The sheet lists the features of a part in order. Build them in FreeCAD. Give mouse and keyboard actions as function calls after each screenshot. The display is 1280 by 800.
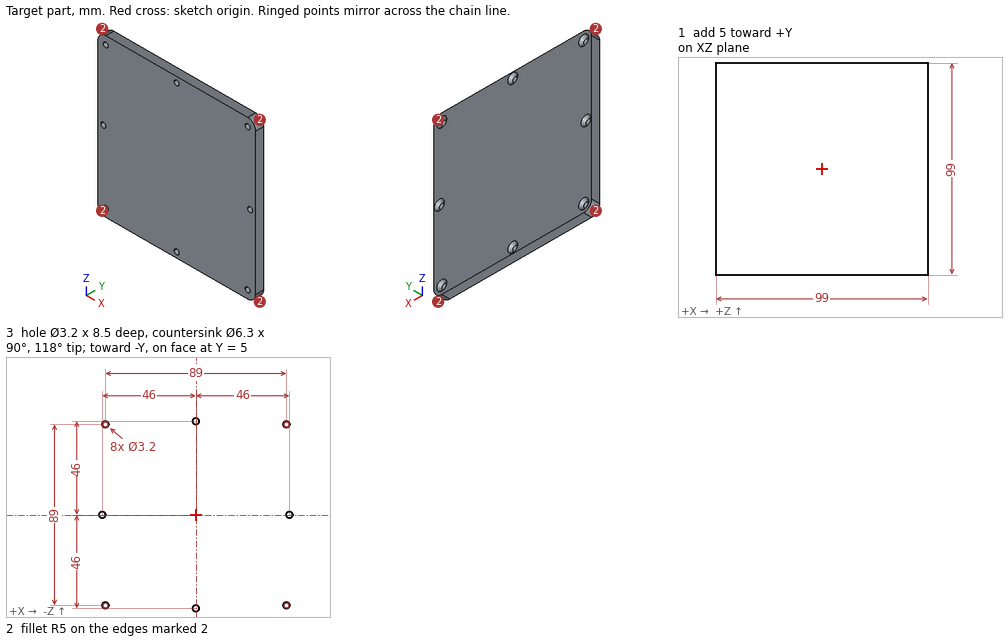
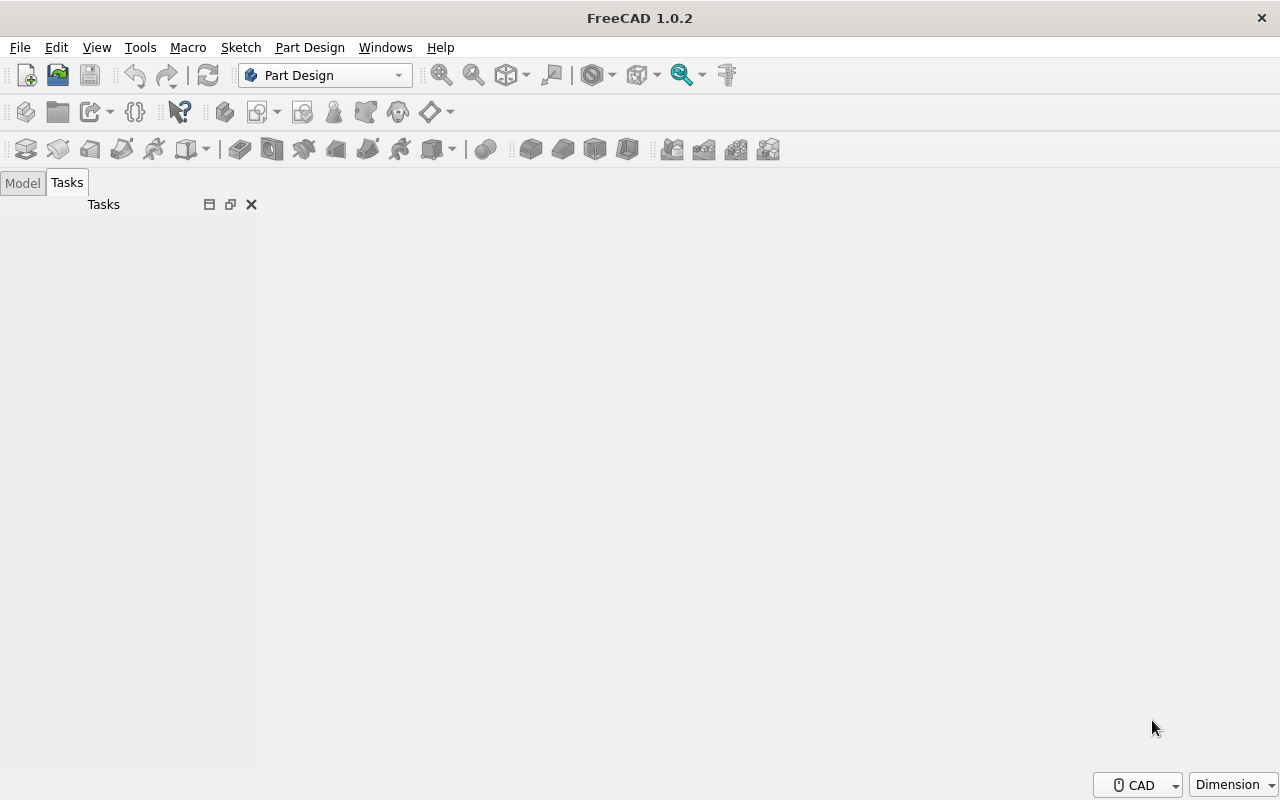
click(26, 76)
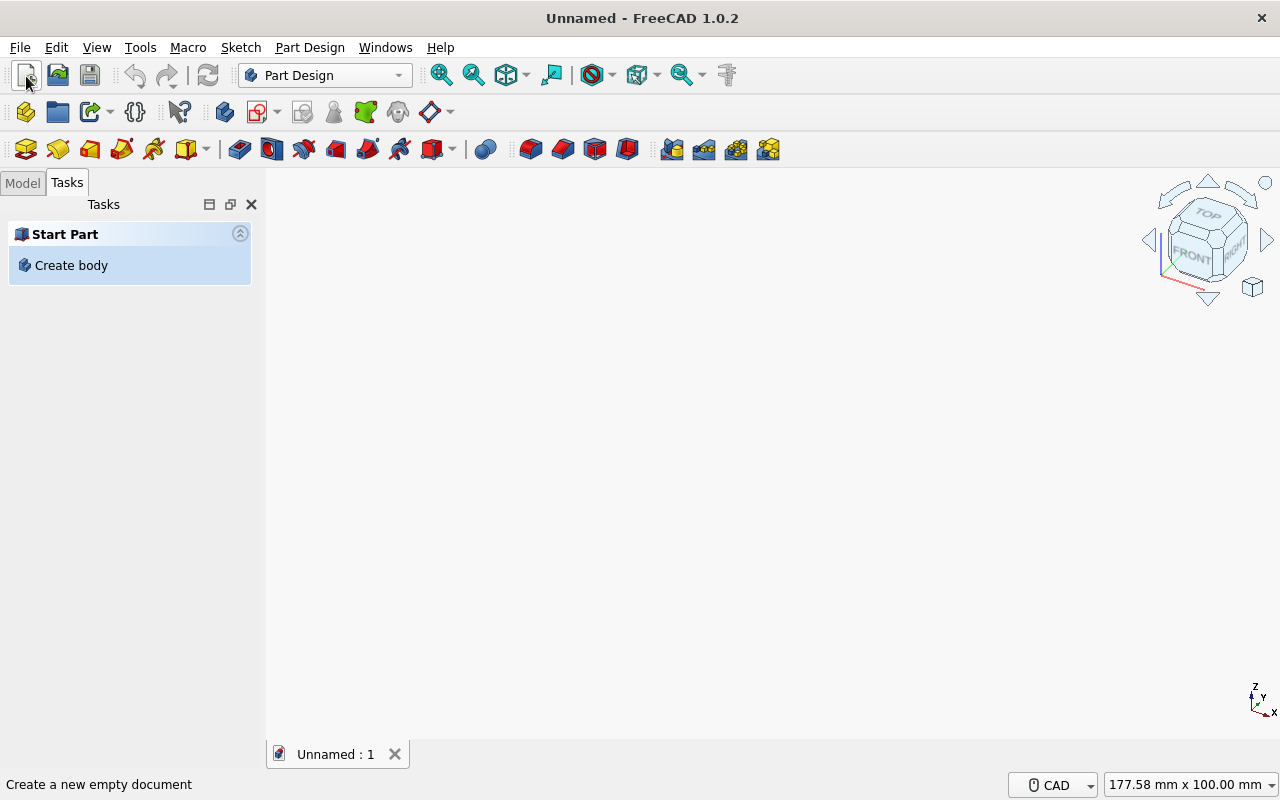
click(258, 112)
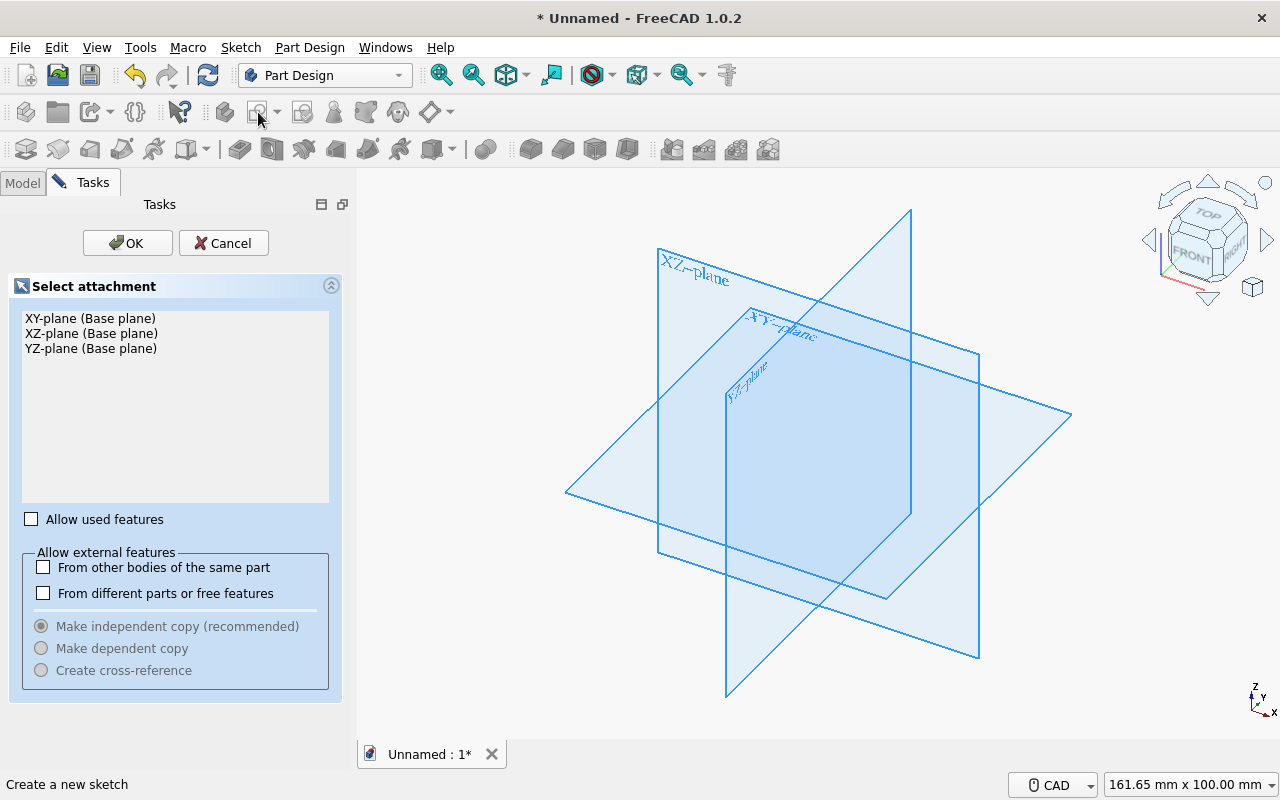
click(82, 334)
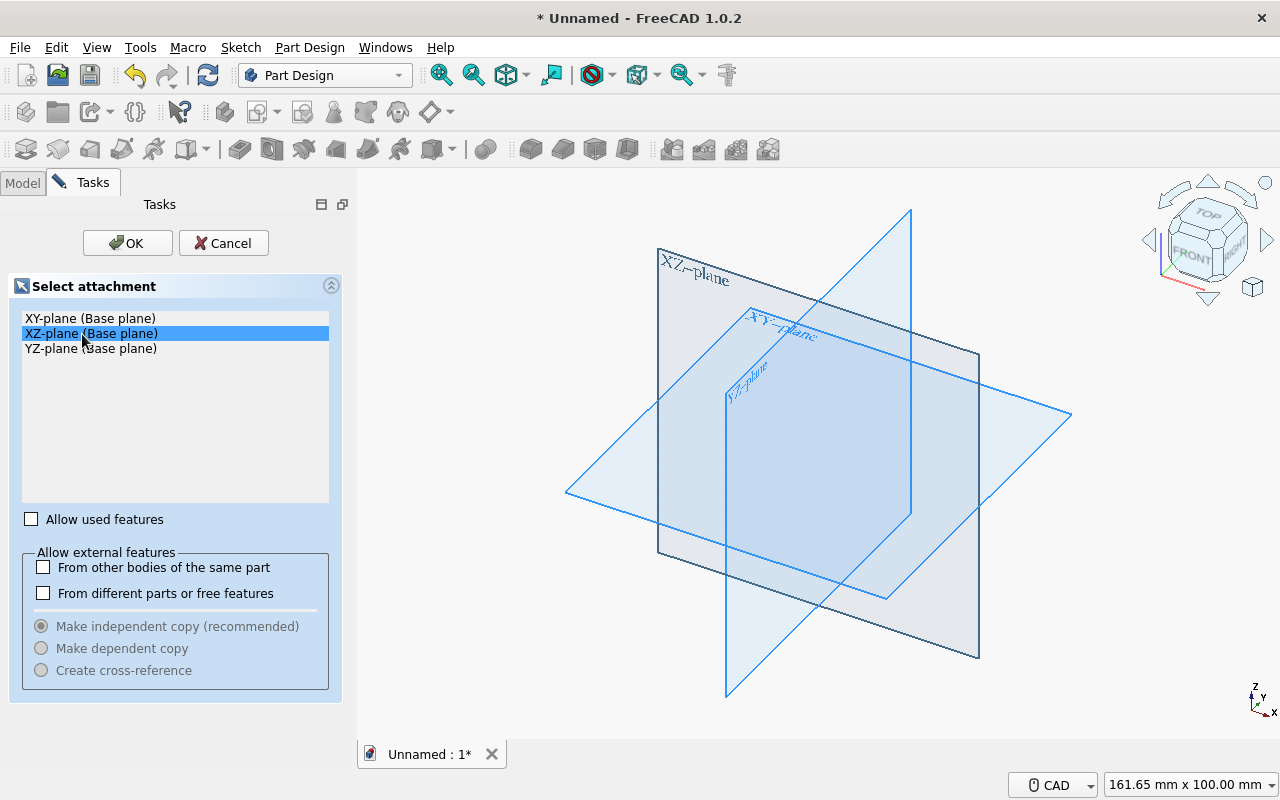
click(128, 243)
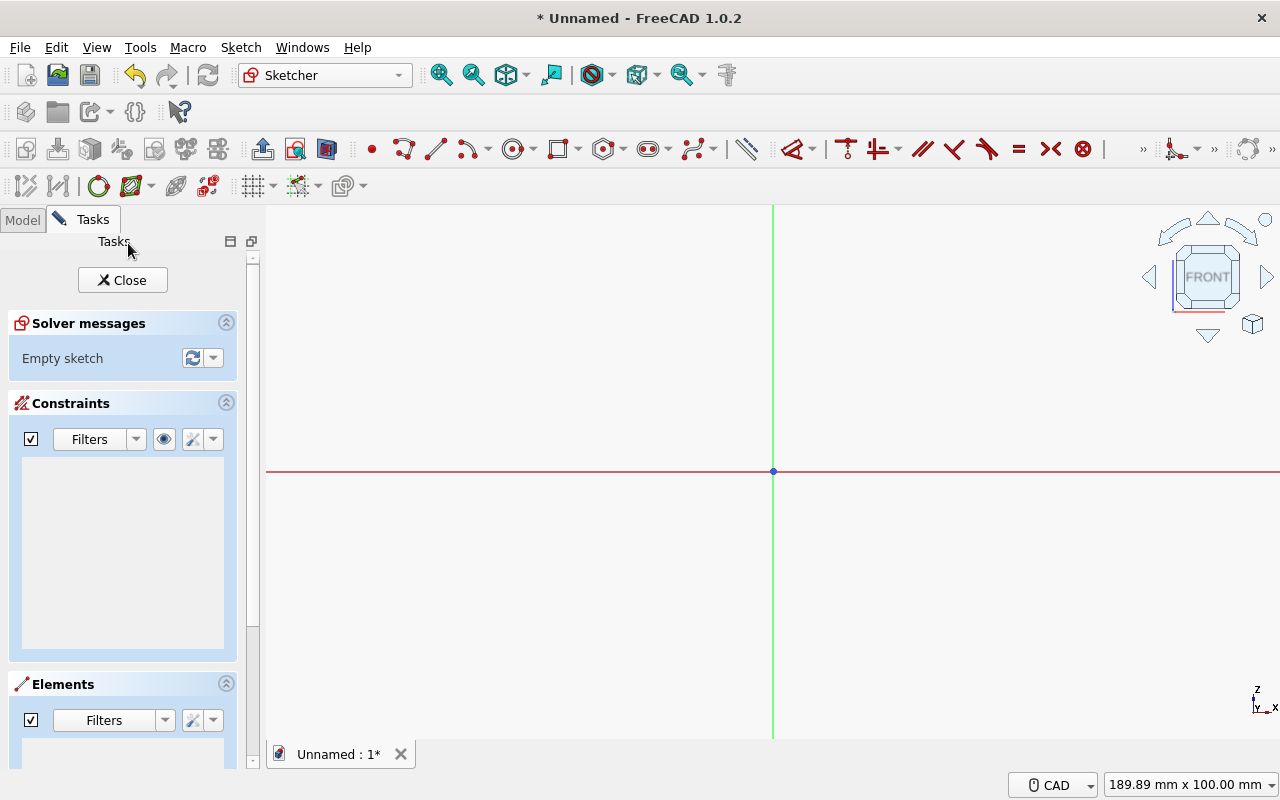
scroll(565, 472, down, 2)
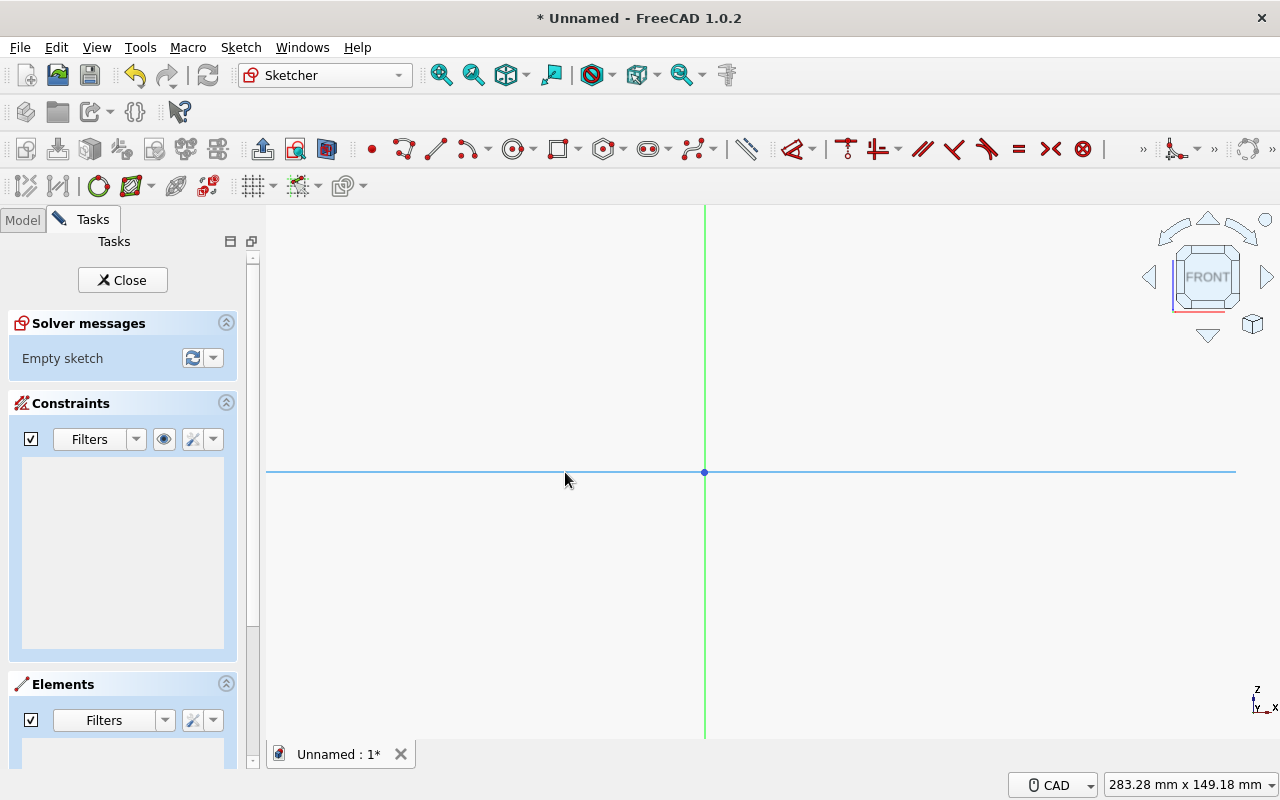
click(580, 150)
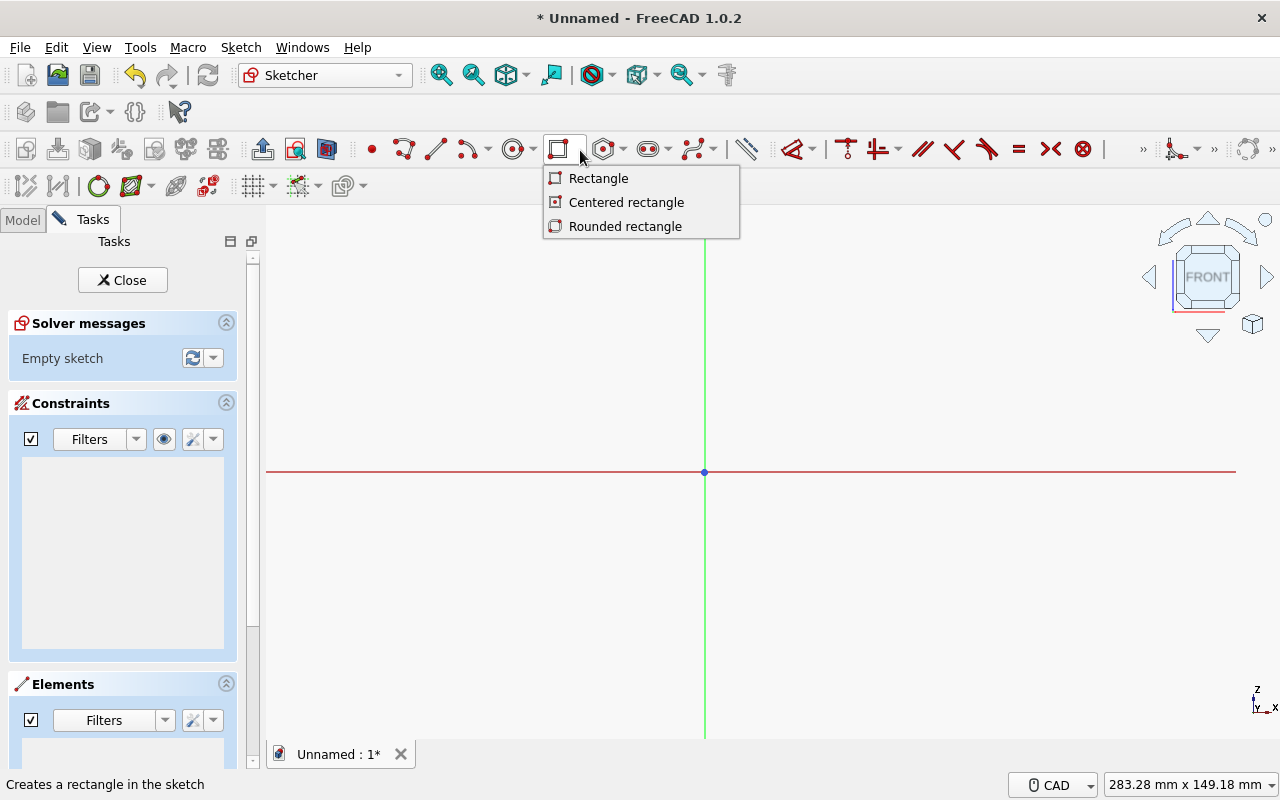
click(642, 202)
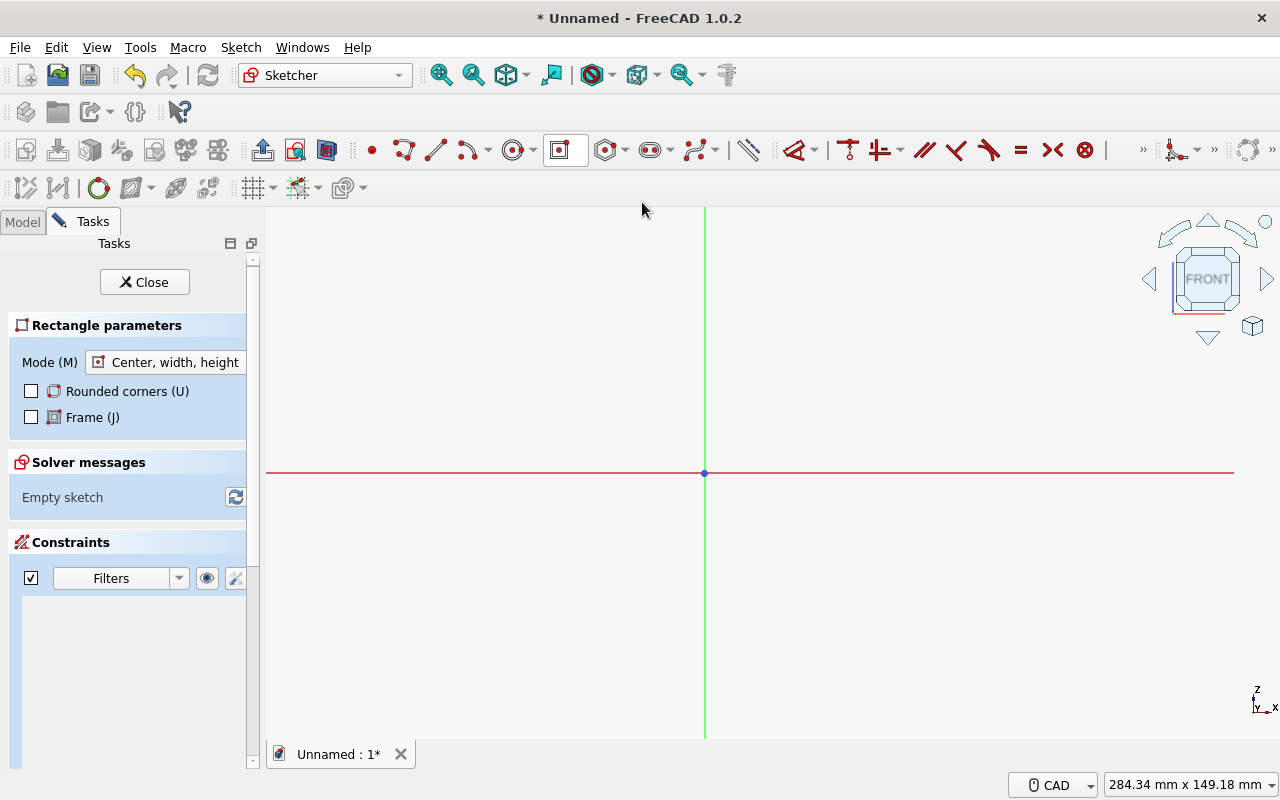
click(705, 473)
move(881, 297)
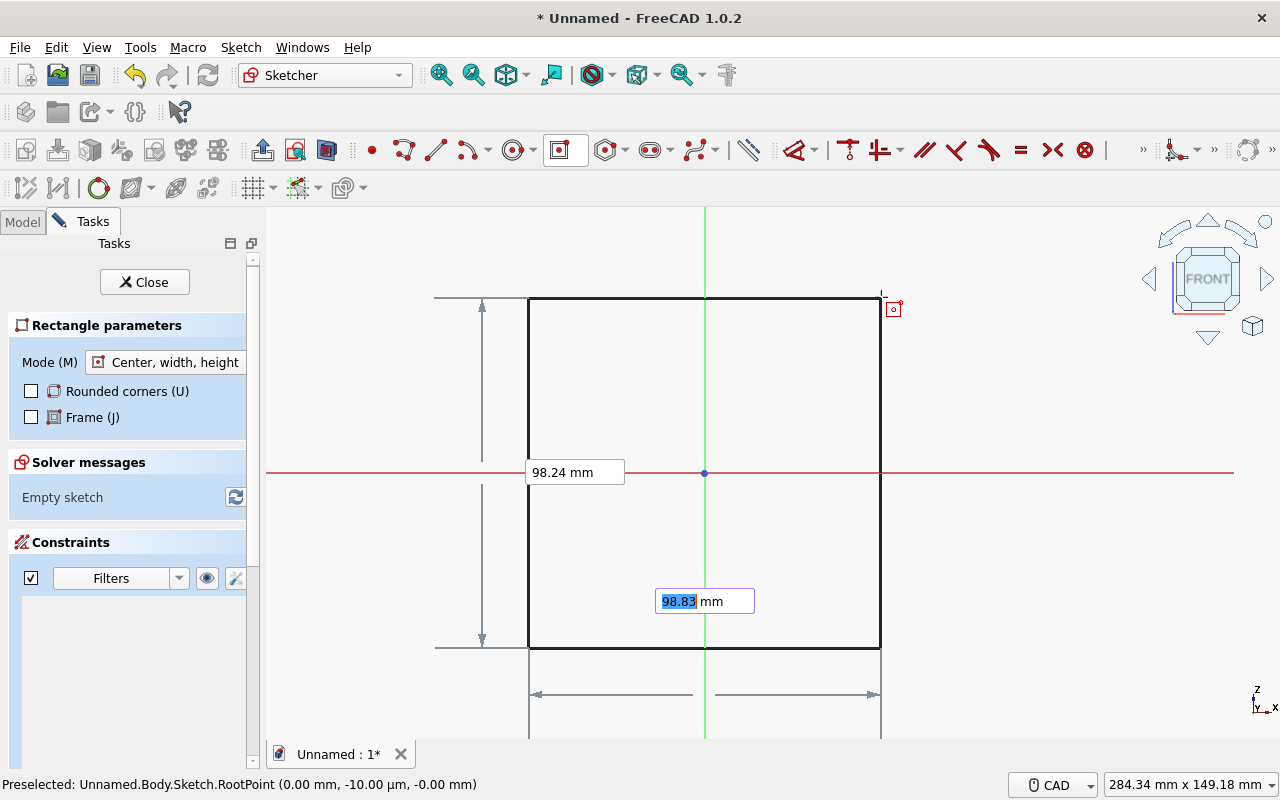
text(99)
key(Tab)
text(99)
key(Return)
key(Escape)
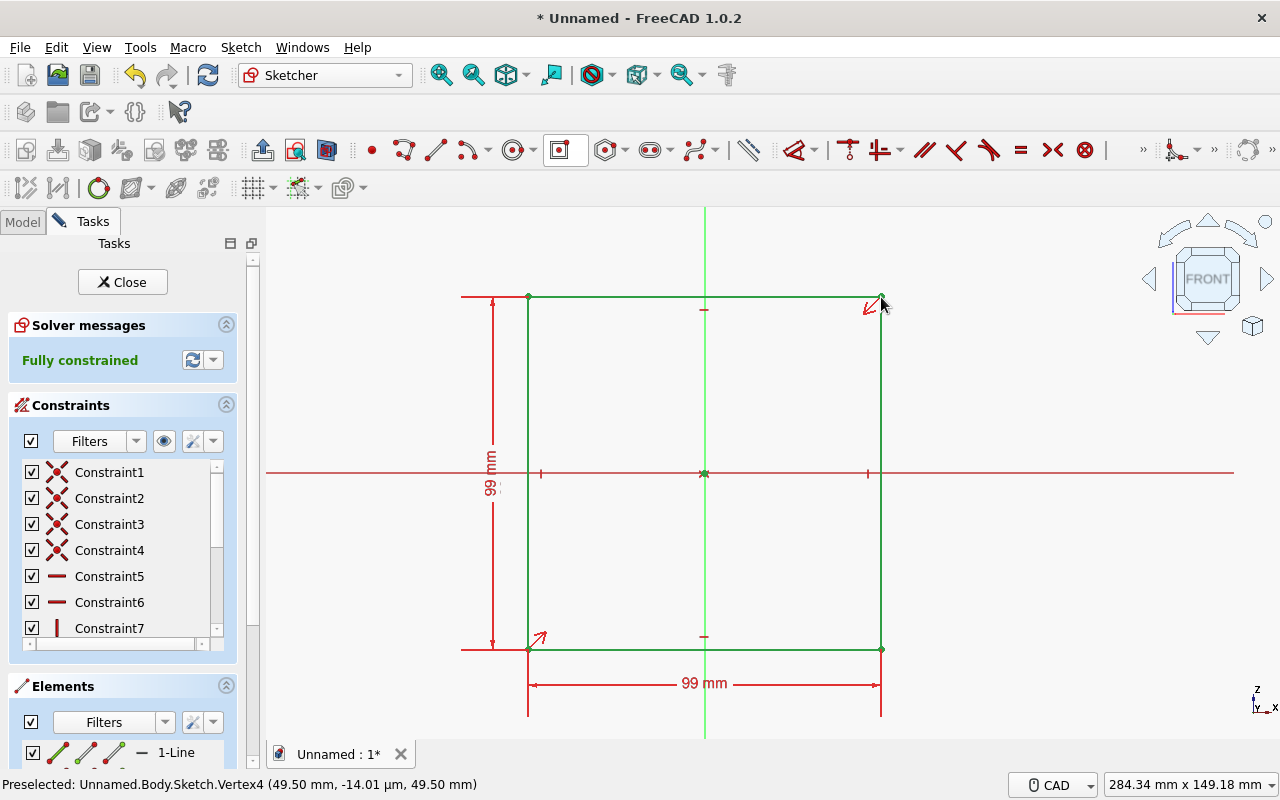
click(123, 282)